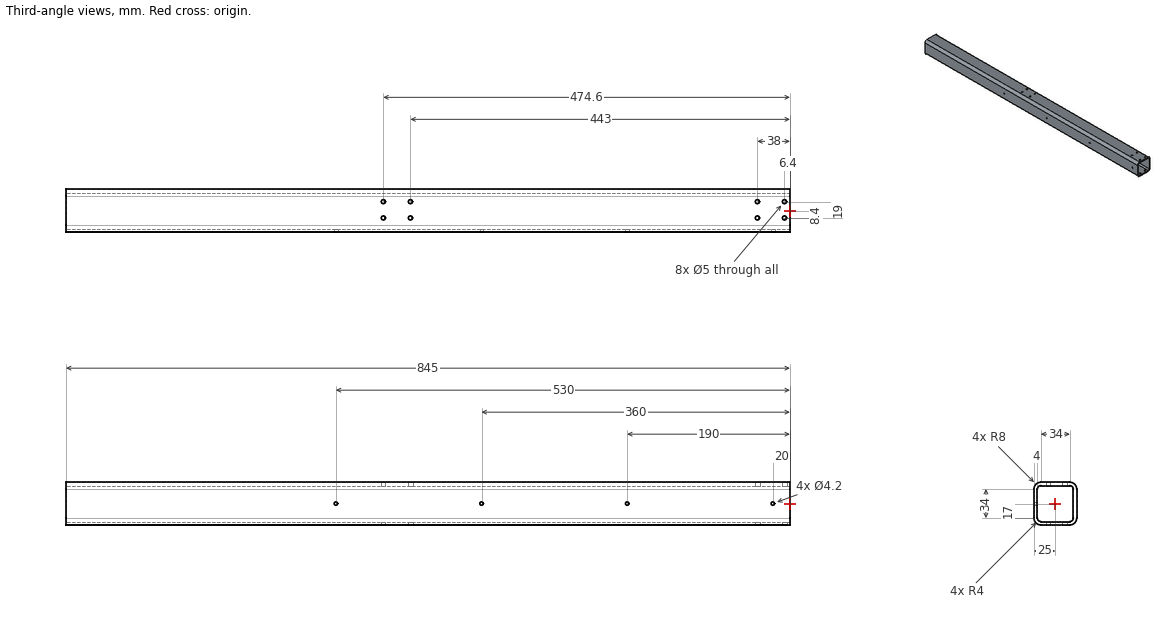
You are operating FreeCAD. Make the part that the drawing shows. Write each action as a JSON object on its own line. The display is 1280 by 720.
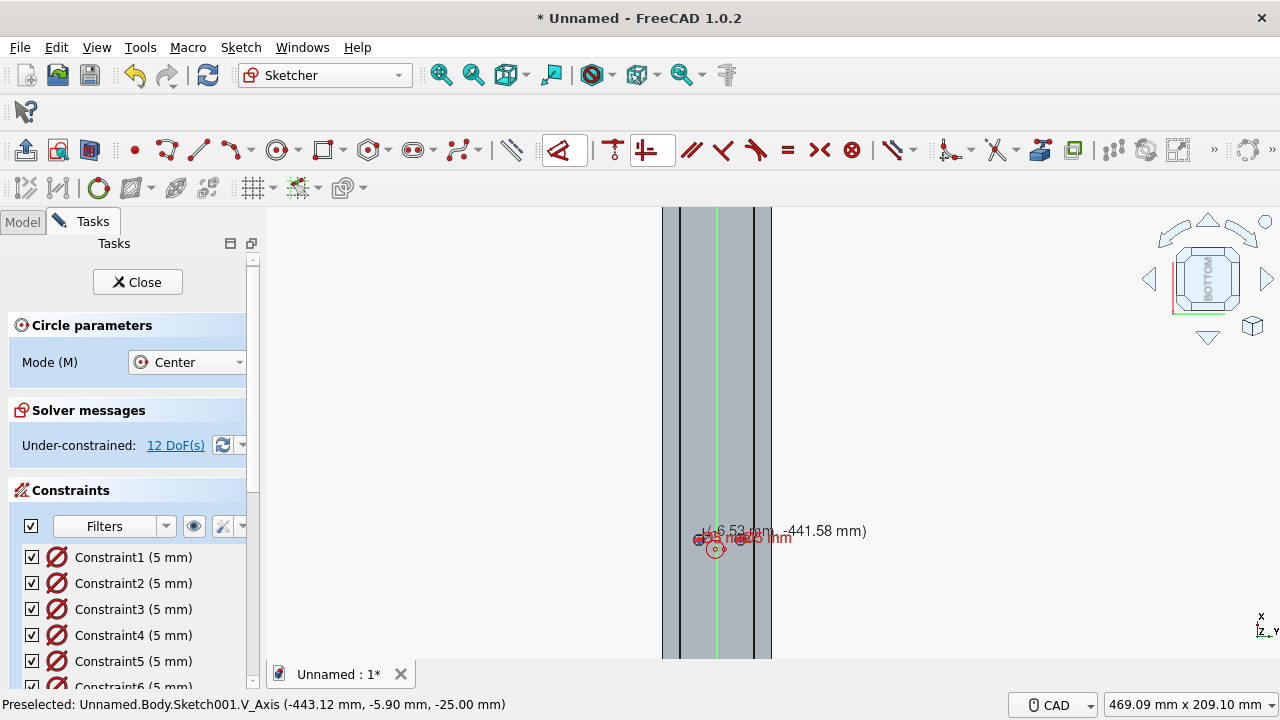
{"action": "scroll", "coordinate": [740, 607], "scroll_direction": "up", "scroll_amount": 8}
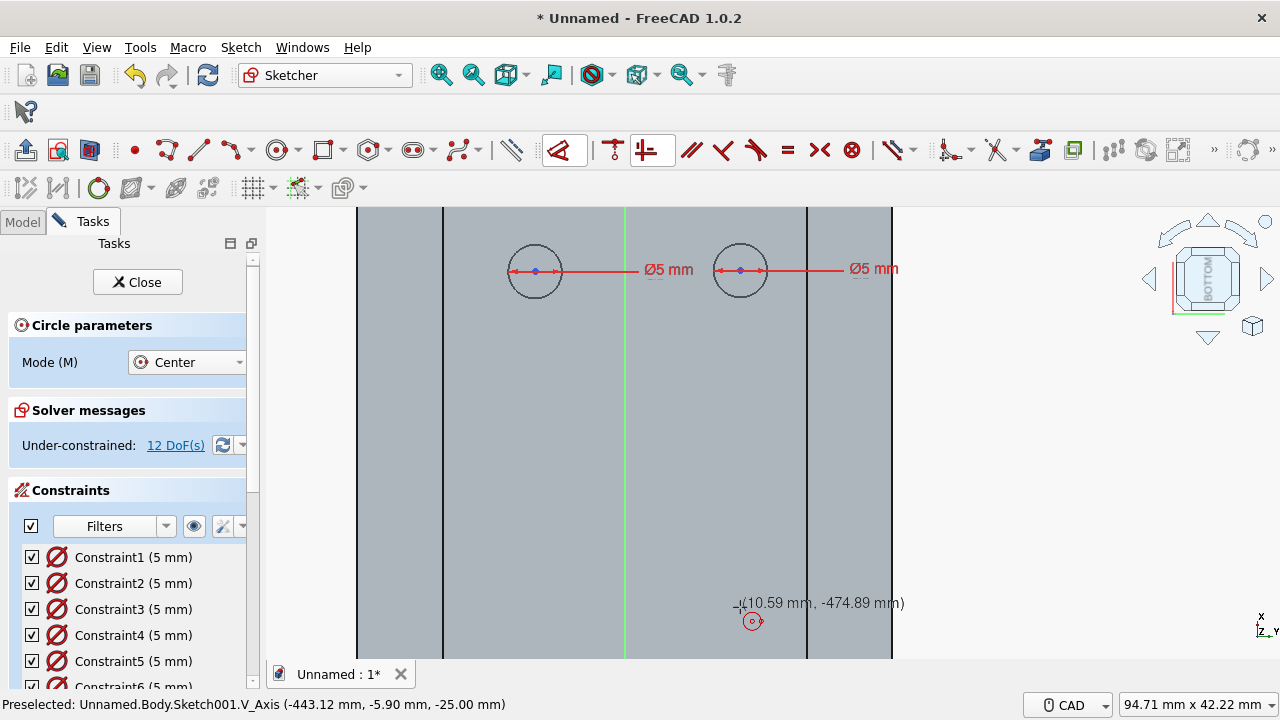
{"action": "scroll", "coordinate": [708, 556], "scroll_direction": "down", "scroll_amount": 15}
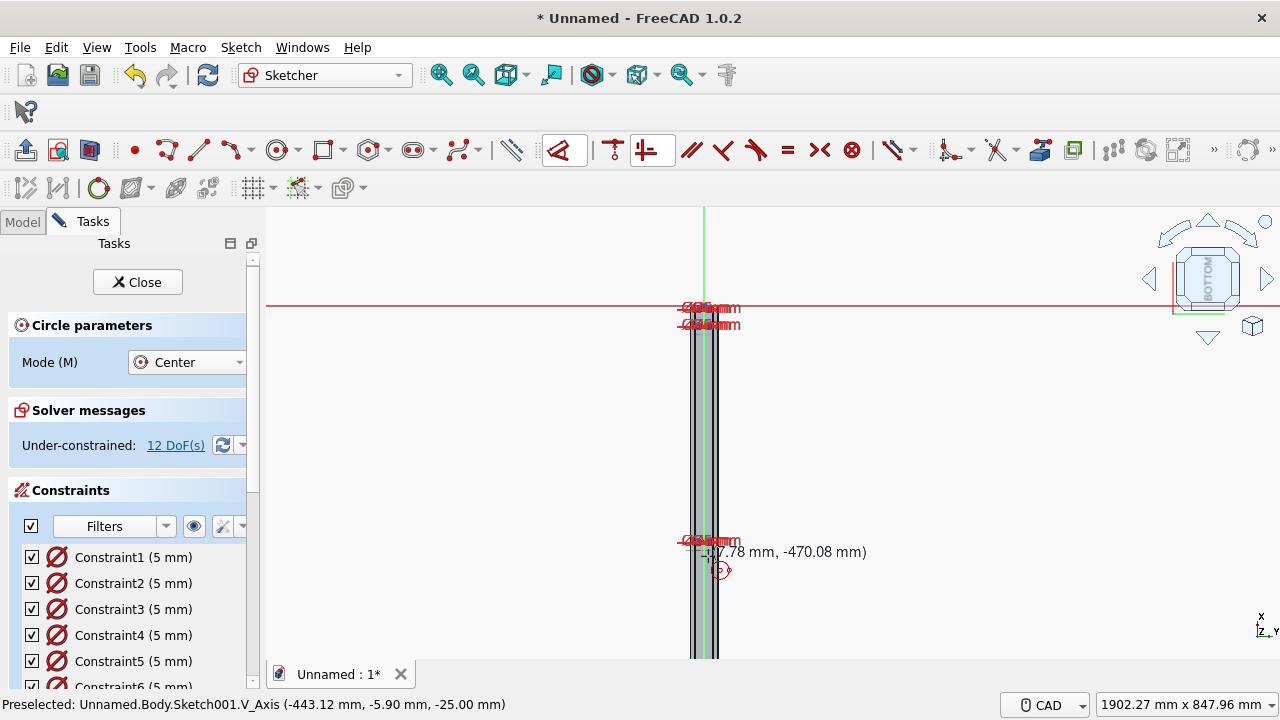
{"action": "scroll", "coordinate": [710, 559], "scroll_direction": "up", "scroll_amount": 6}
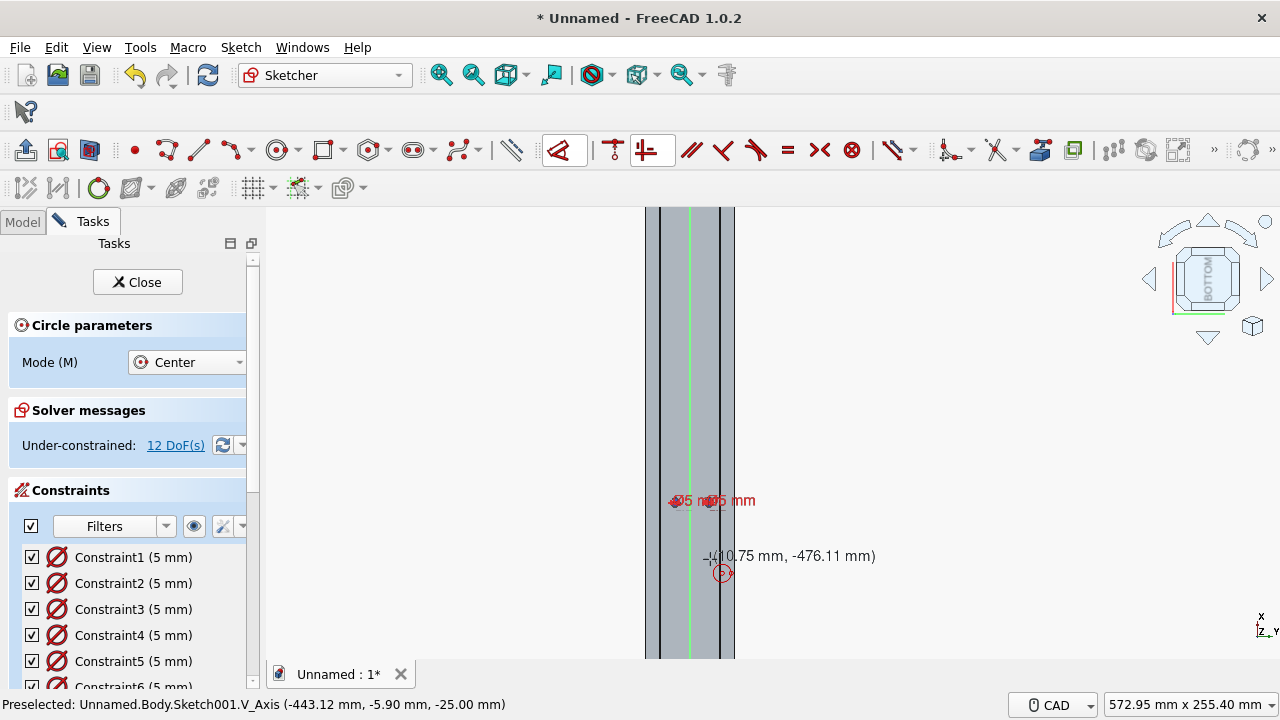
{"action": "left_click", "coordinate": [709, 558]}
{"action": "mouse_move", "coordinate": [712, 555]}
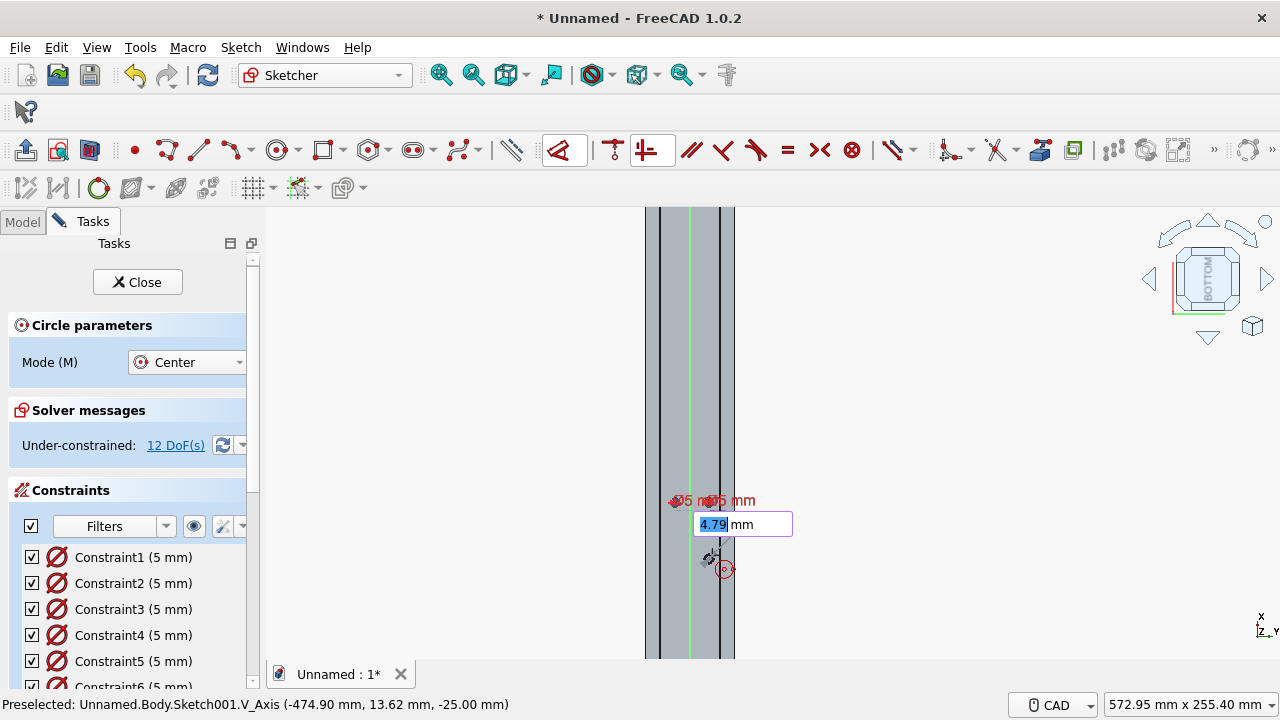
{"action": "type", "text": "5"}
{"action": "key", "text": "Return"}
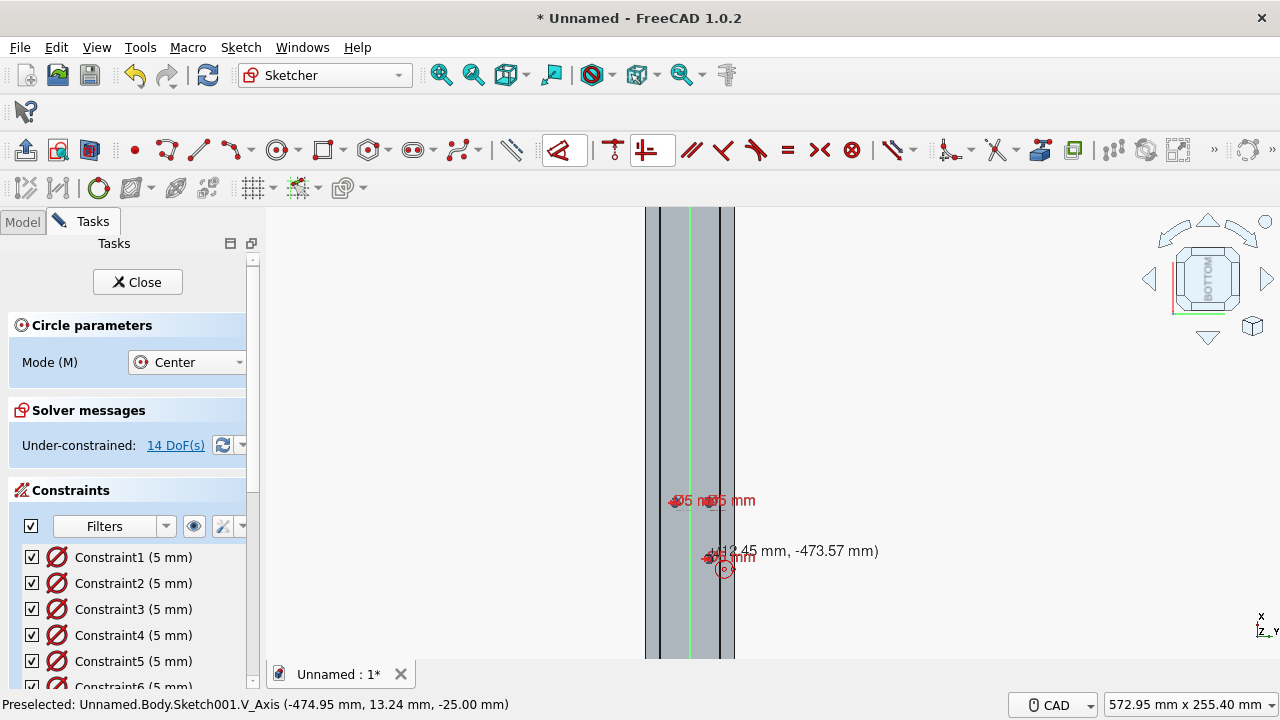
{"action": "scroll", "coordinate": [675, 558], "scroll_direction": "up", "scroll_amount": 9}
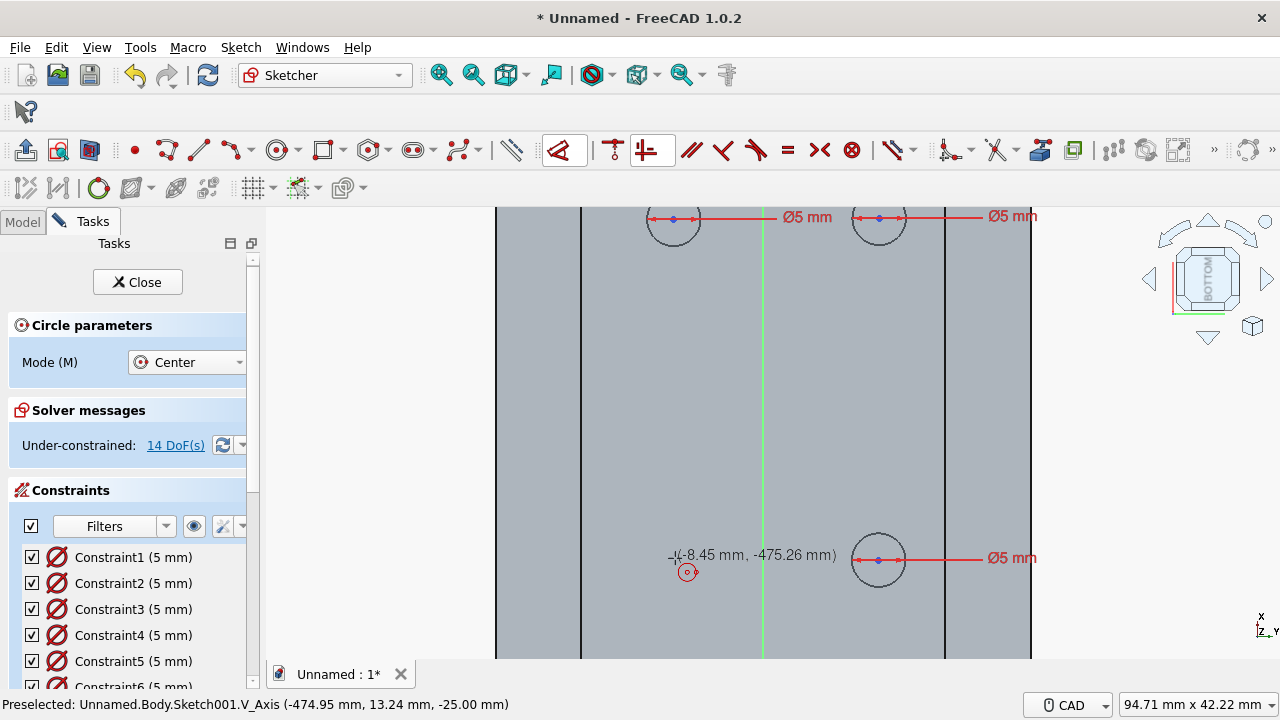
{"action": "scroll", "coordinate": [701, 559], "scroll_direction": "down", "scroll_amount": 15}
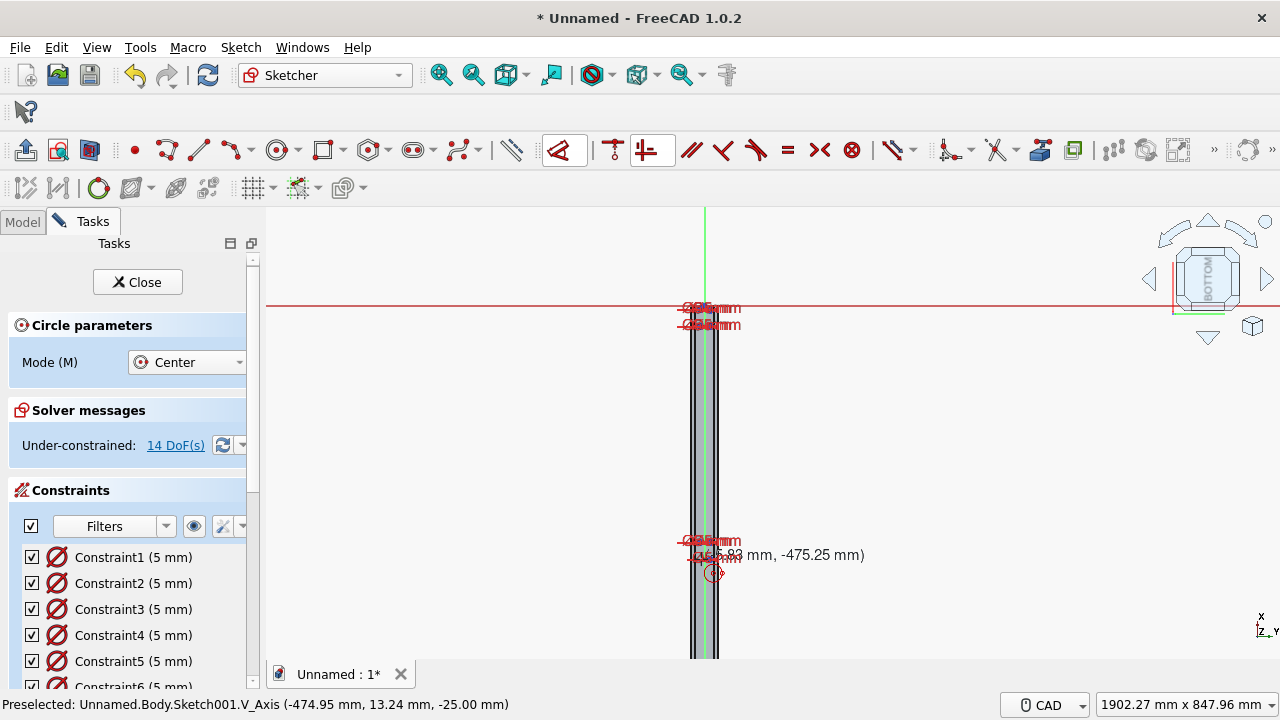
{"action": "scroll", "coordinate": [700, 559], "scroll_direction": "up", "scroll_amount": 7}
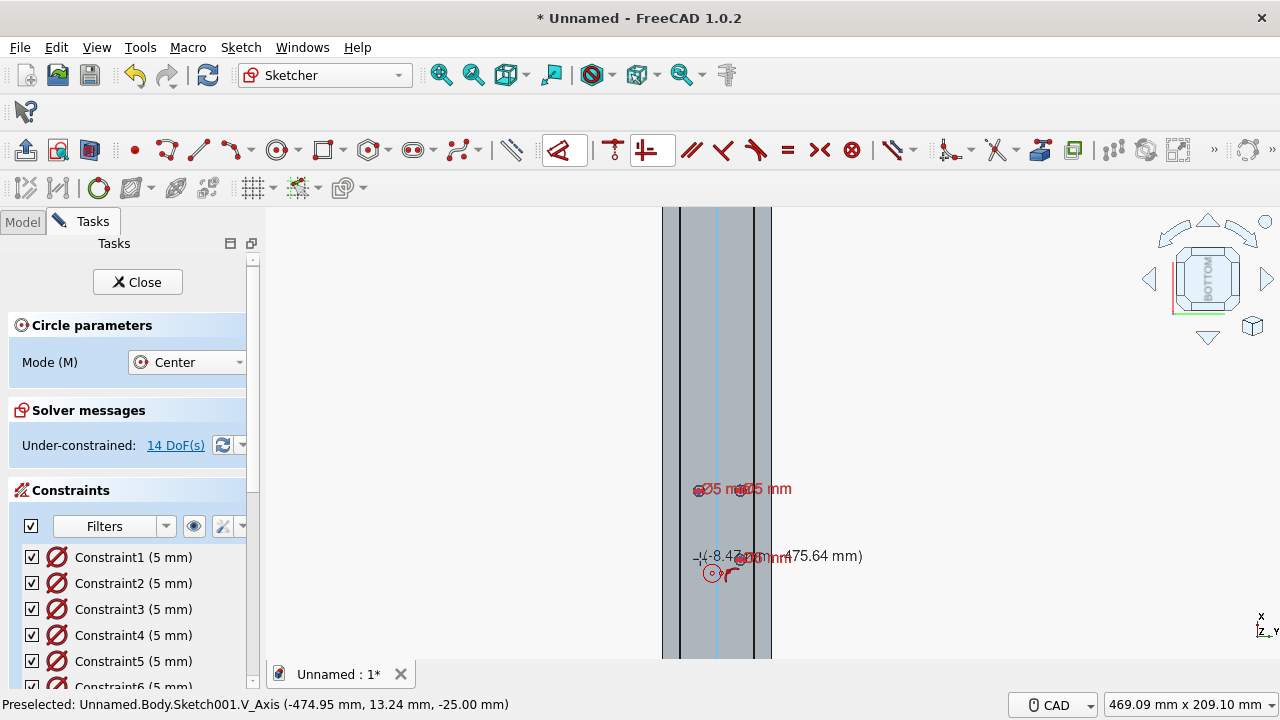
{"action": "left_click", "coordinate": [699, 558]}
{"action": "mouse_move", "coordinate": [703, 555]}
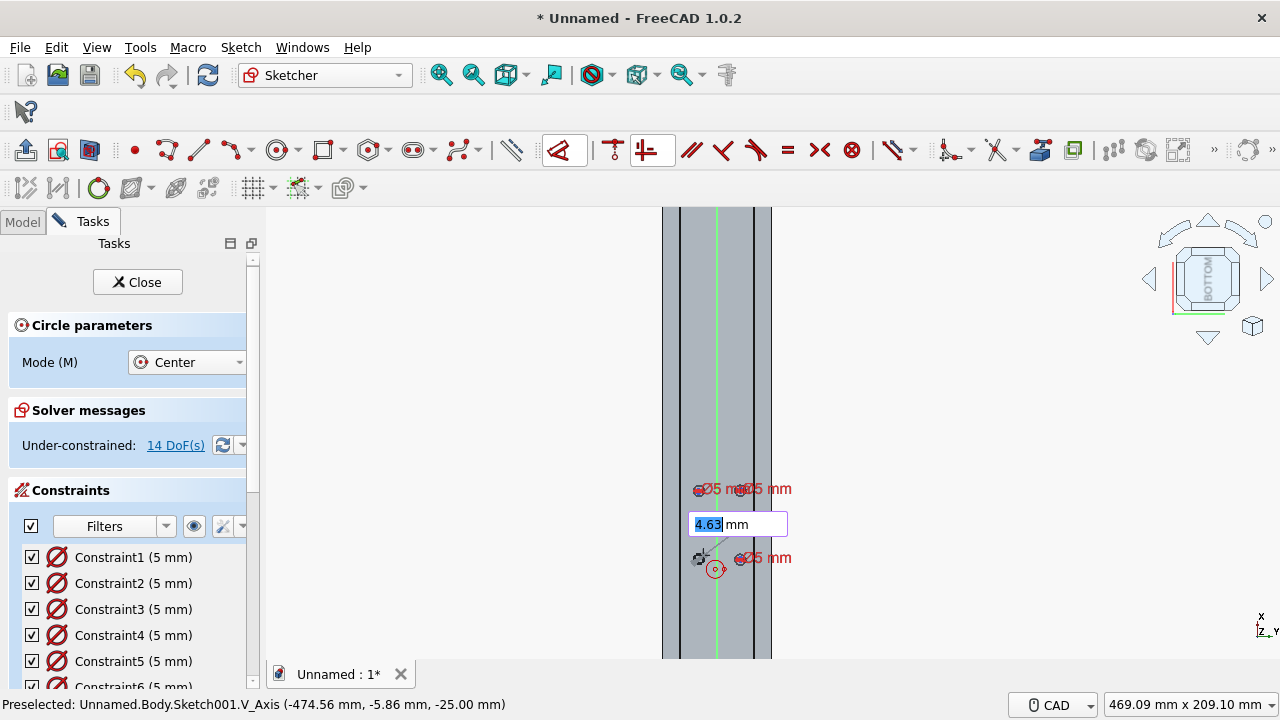
{"action": "type", "text": "5"}
{"action": "key", "text": "Return"}
{"action": "key", "text": "Escape"}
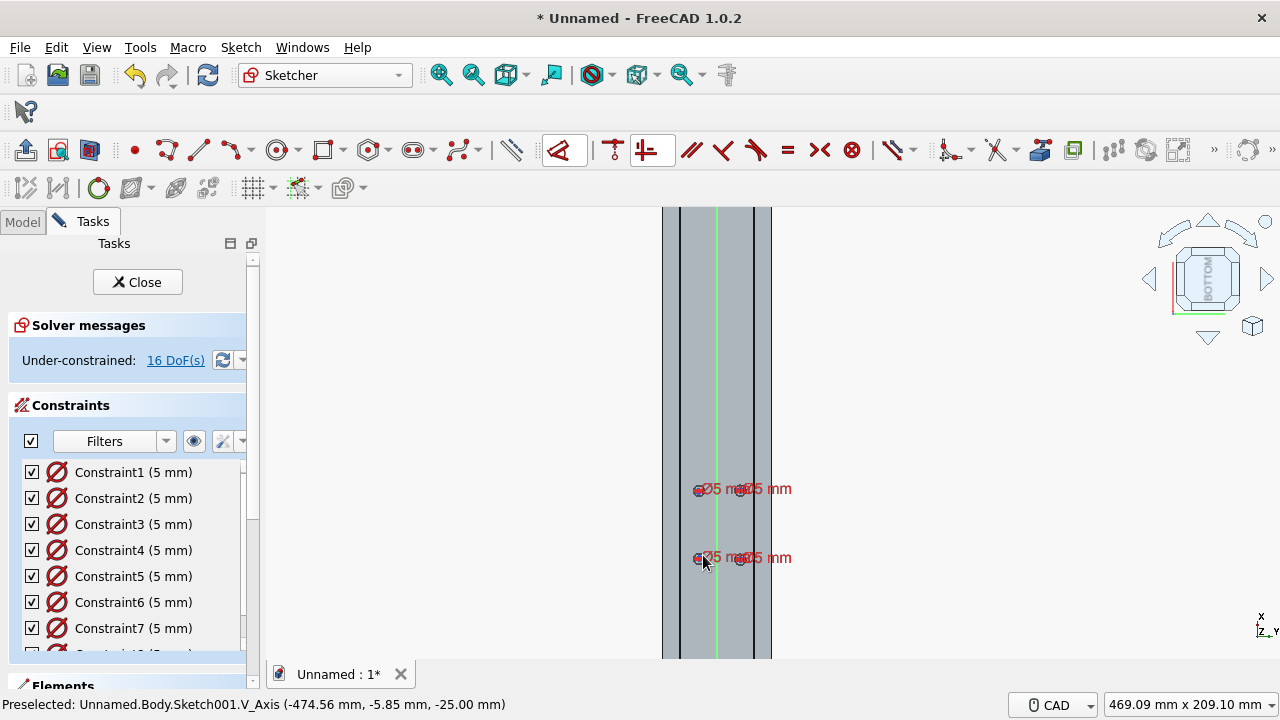
{"action": "scroll", "coordinate": [700, 559], "scroll_direction": "down", "scroll_amount": 7}